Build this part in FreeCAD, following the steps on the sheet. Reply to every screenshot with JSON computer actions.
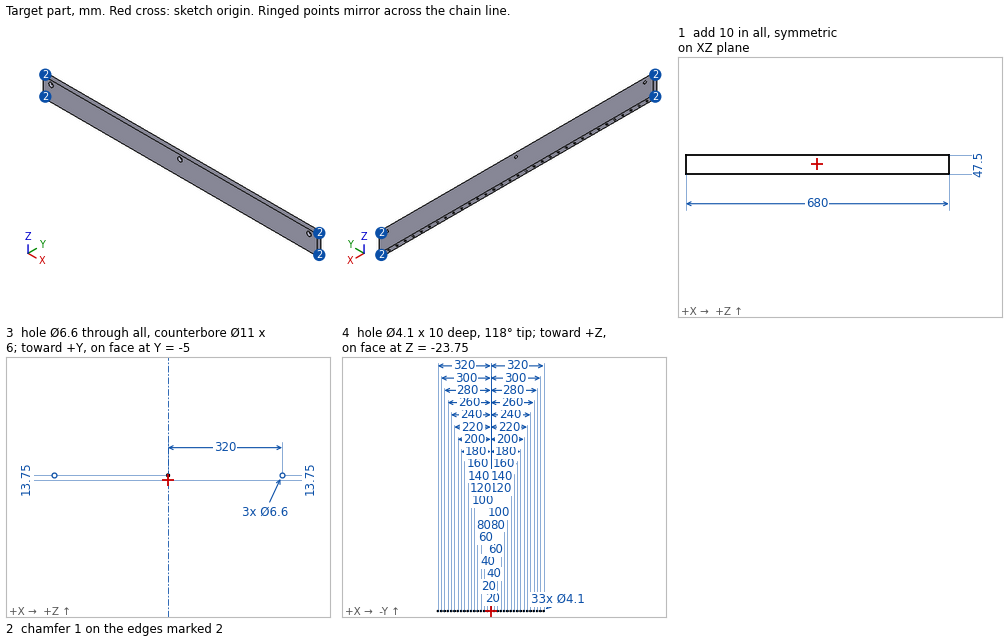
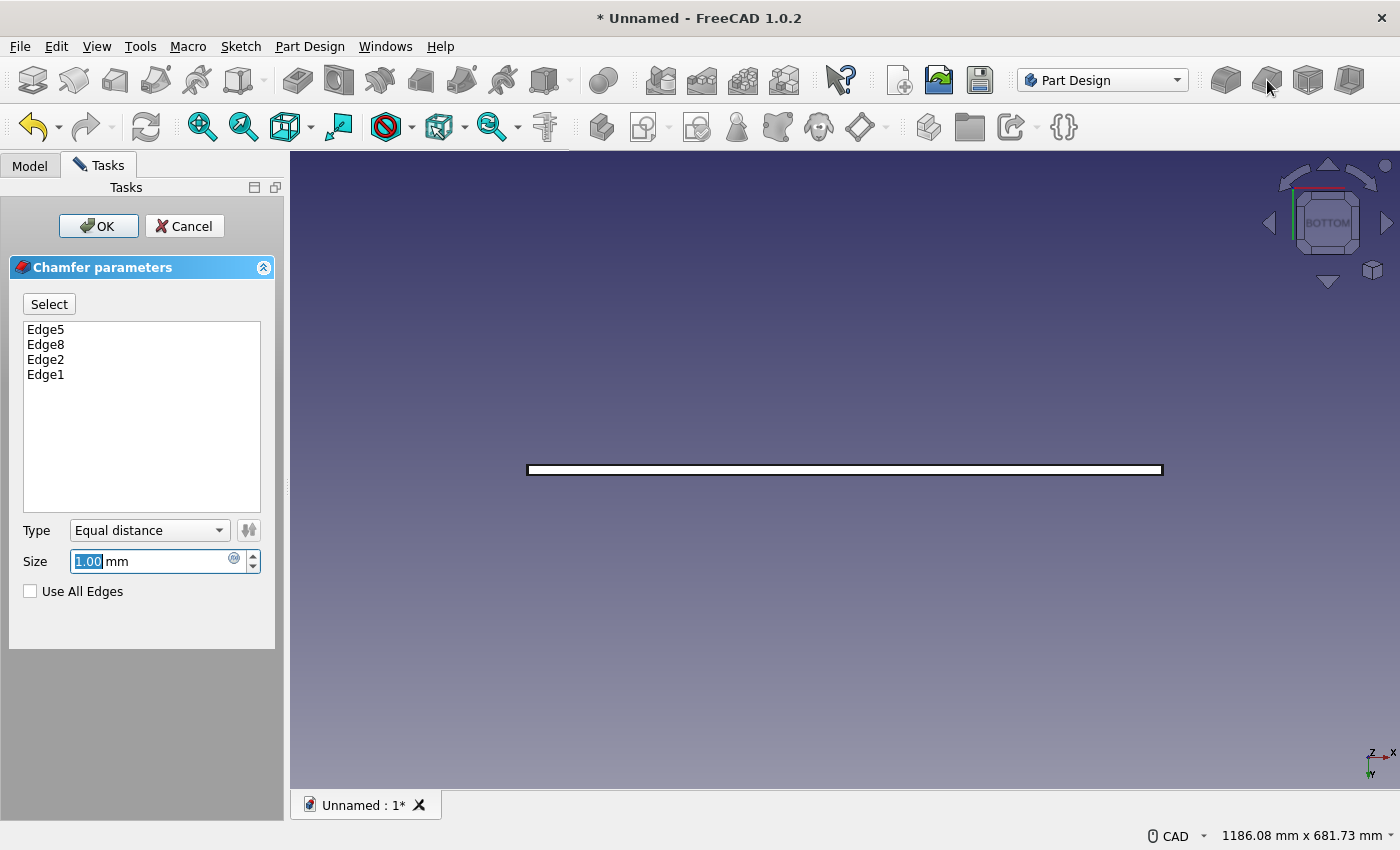
{"action": "type", "text": "1"}
{"action": "key", "text": "Tab"}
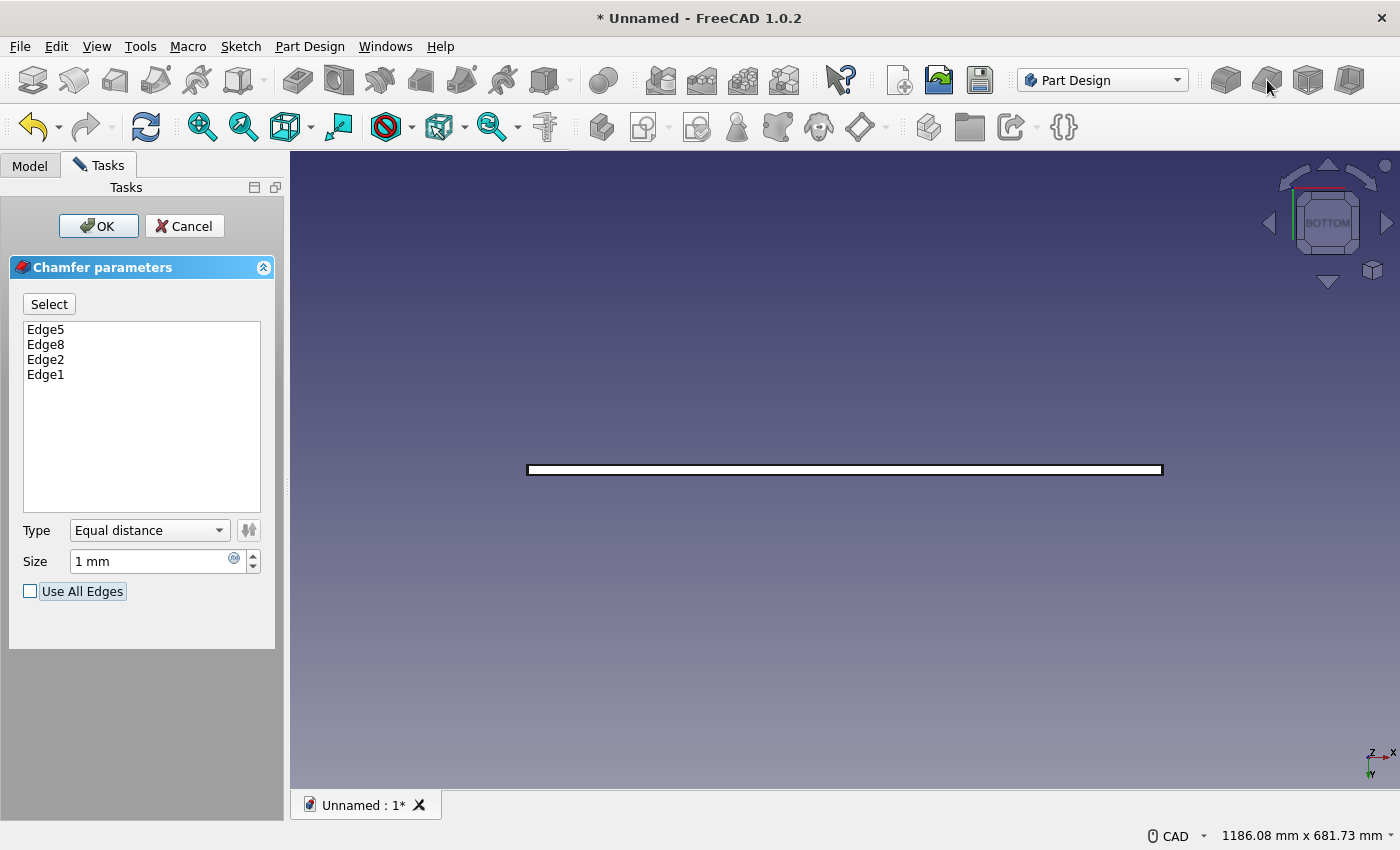
{"action": "left_click", "coordinate": [99, 226]}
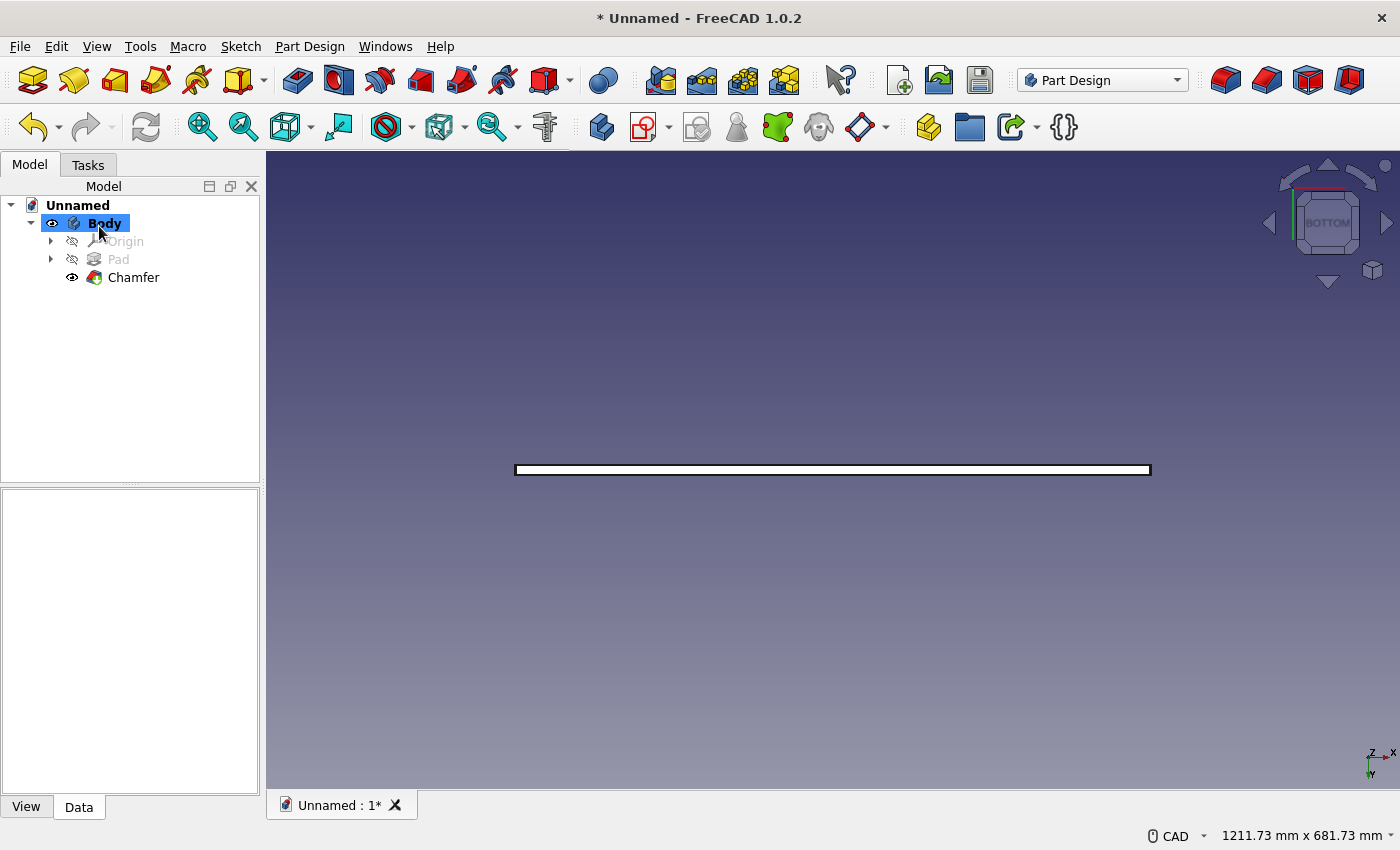
{"action": "key", "text": "0"}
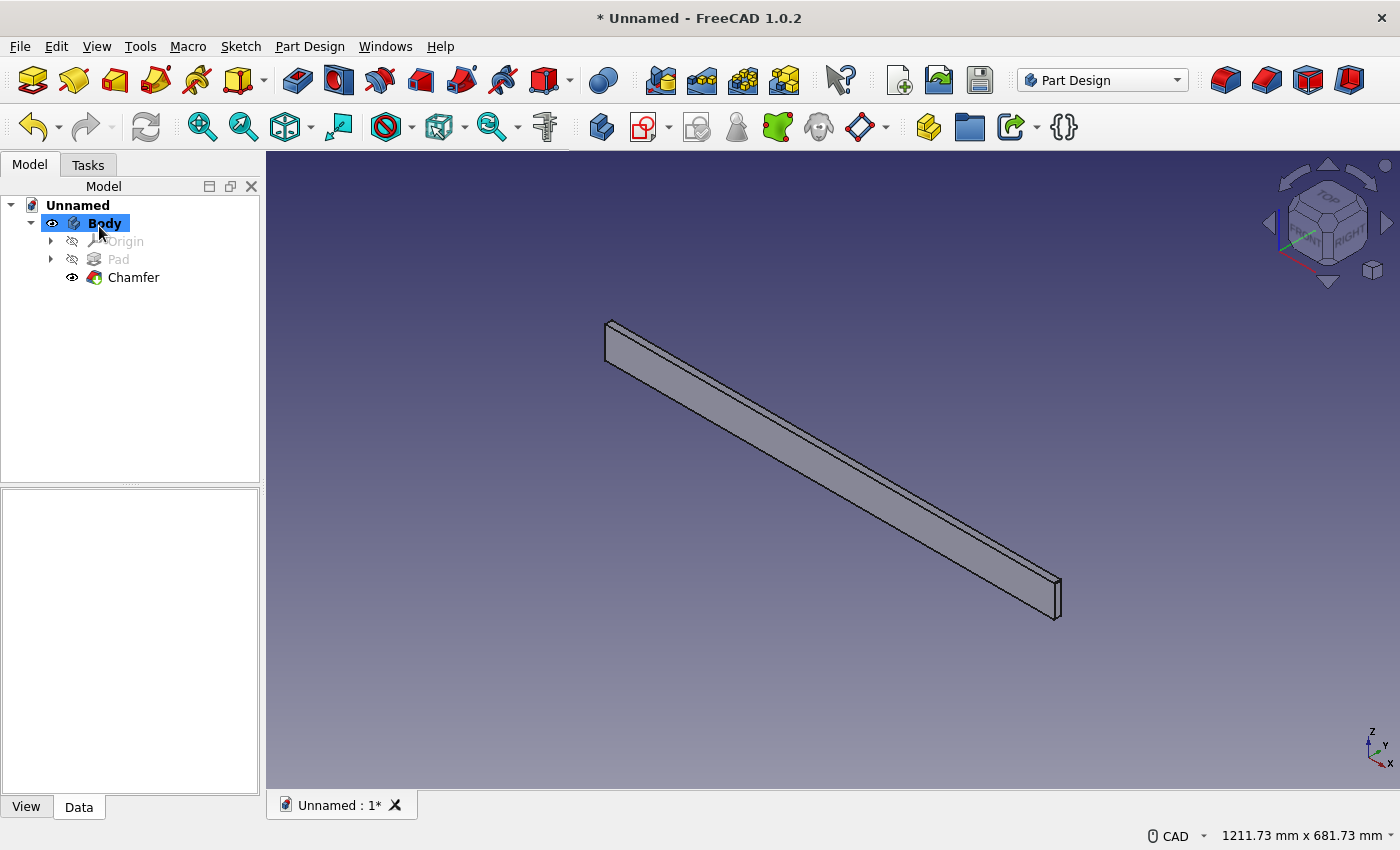
{"action": "left_click", "coordinate": [1023, 582]}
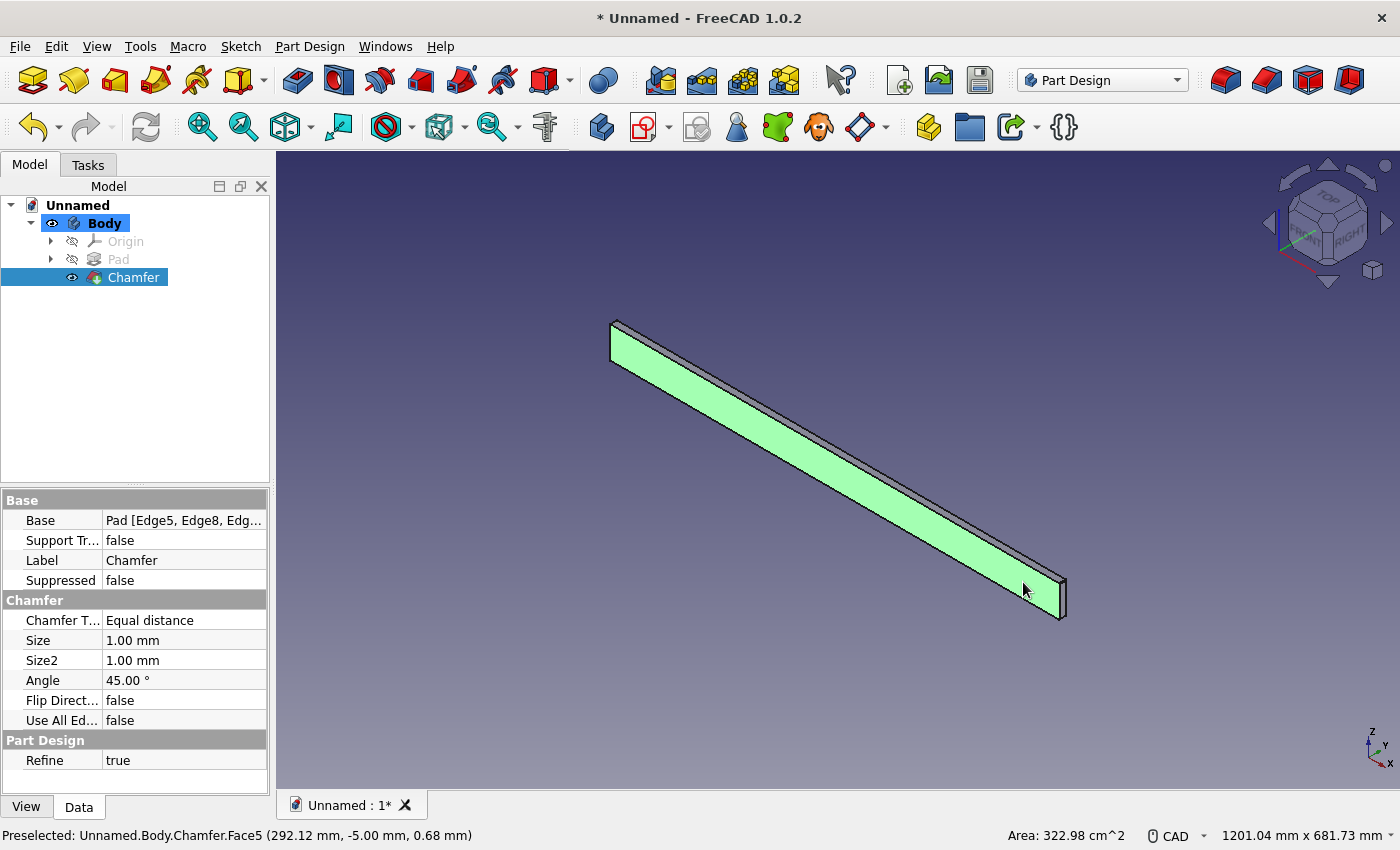
{"action": "left_click", "coordinate": [642, 128]}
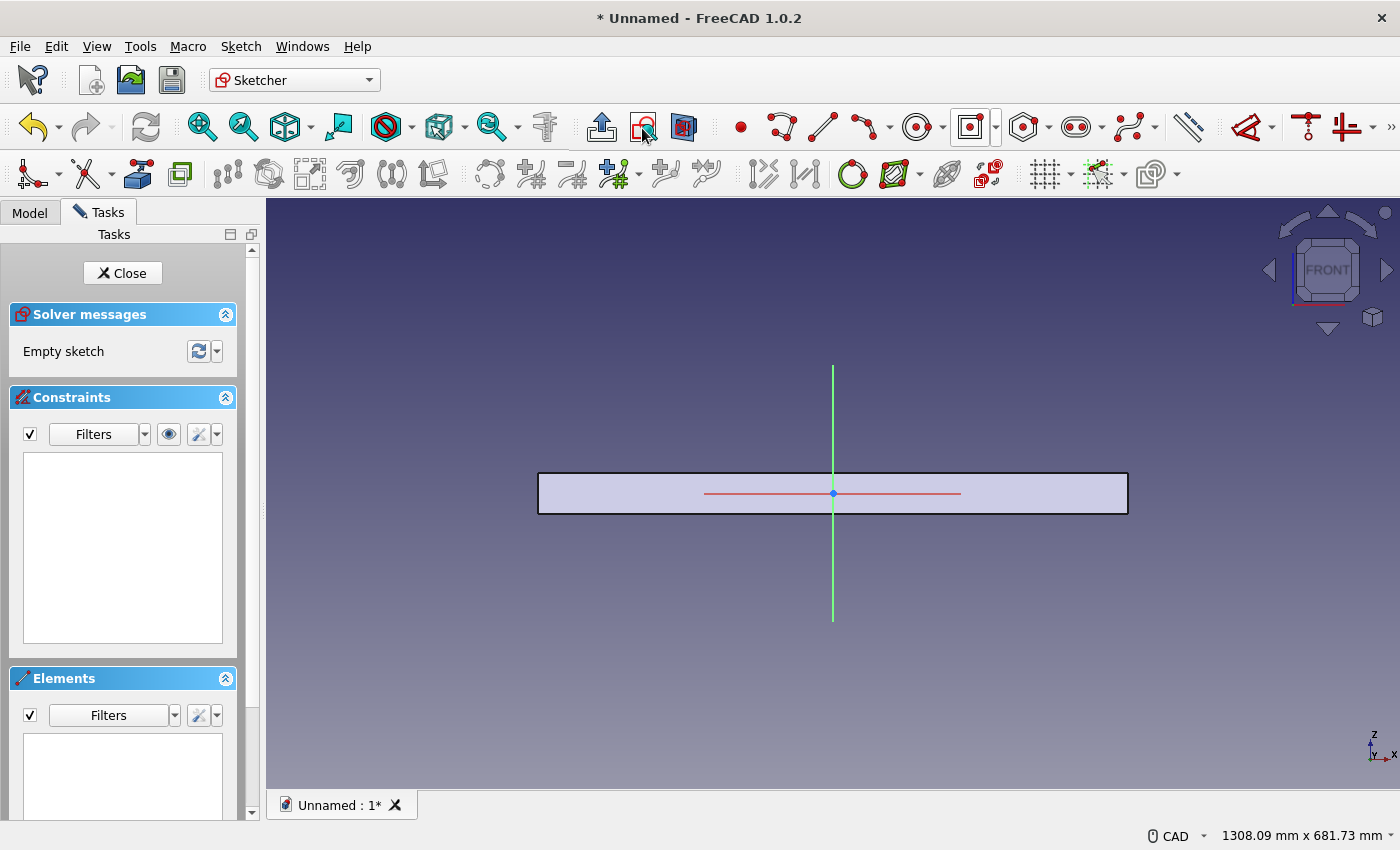
{"action": "left_click", "coordinate": [916, 128]}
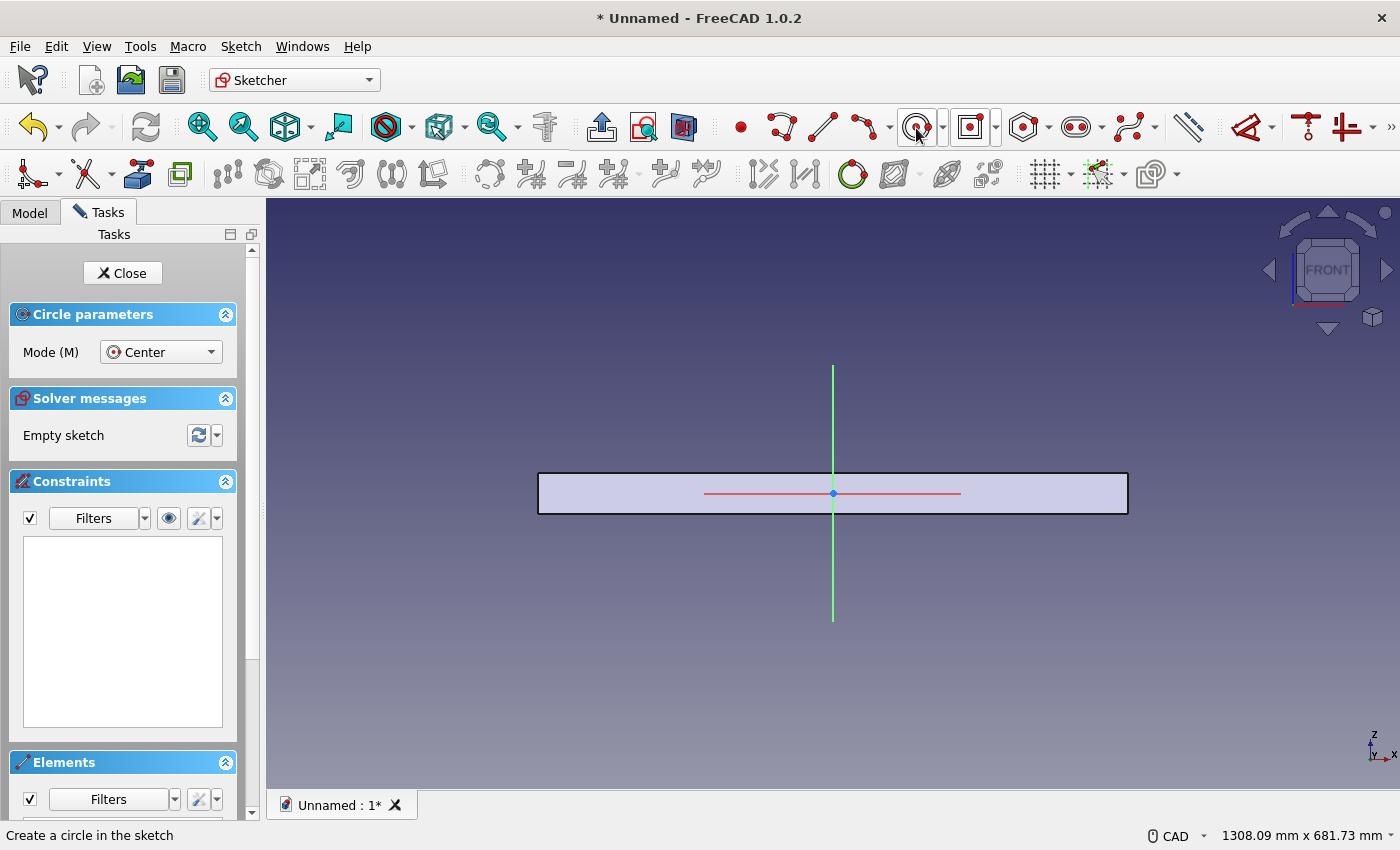
{"action": "scroll", "coordinate": [1110, 482], "scroll_direction": "up", "scroll_amount": 11}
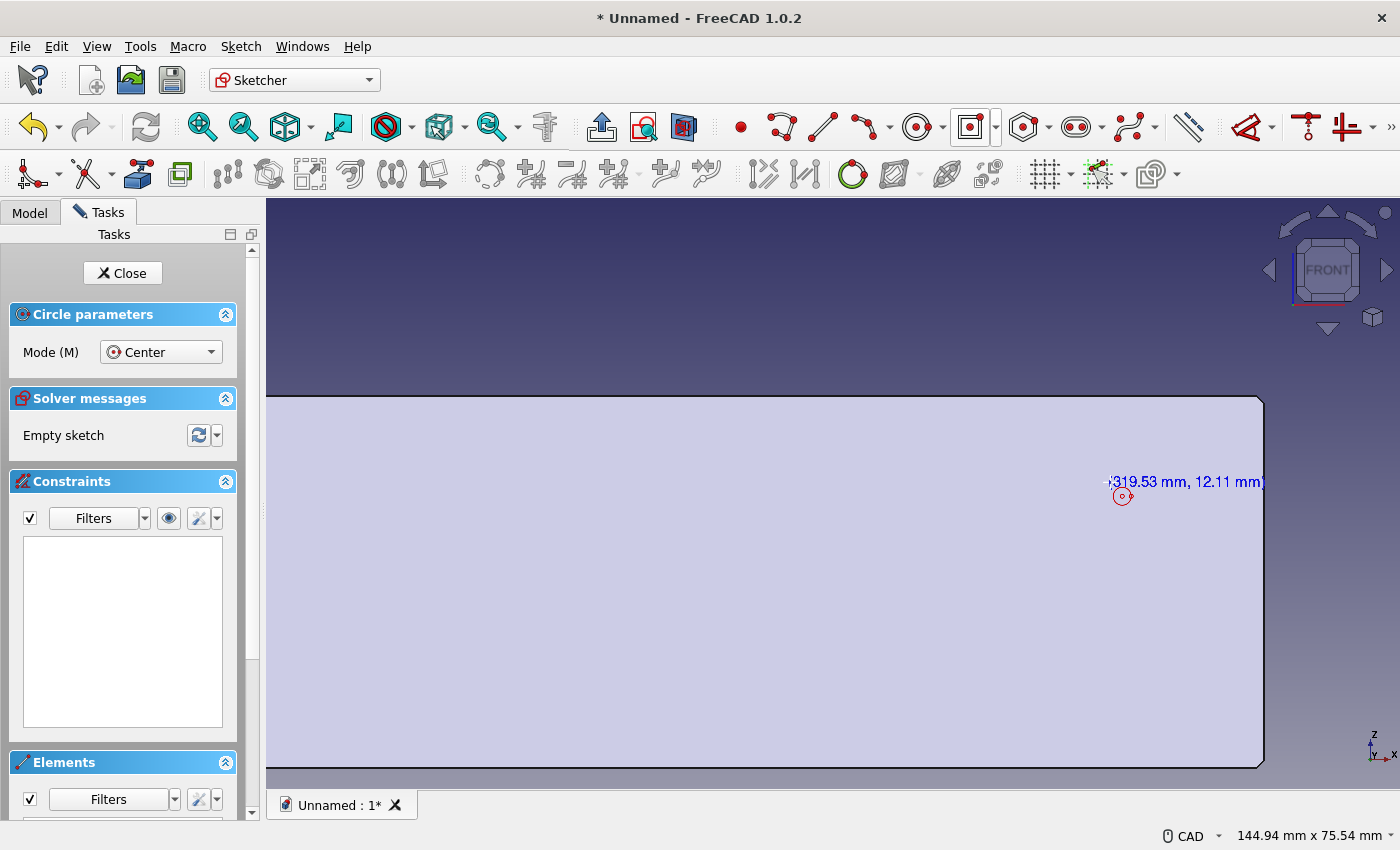
{"action": "scroll", "coordinate": [1103, 490], "scroll_direction": "down", "scroll_amount": 10}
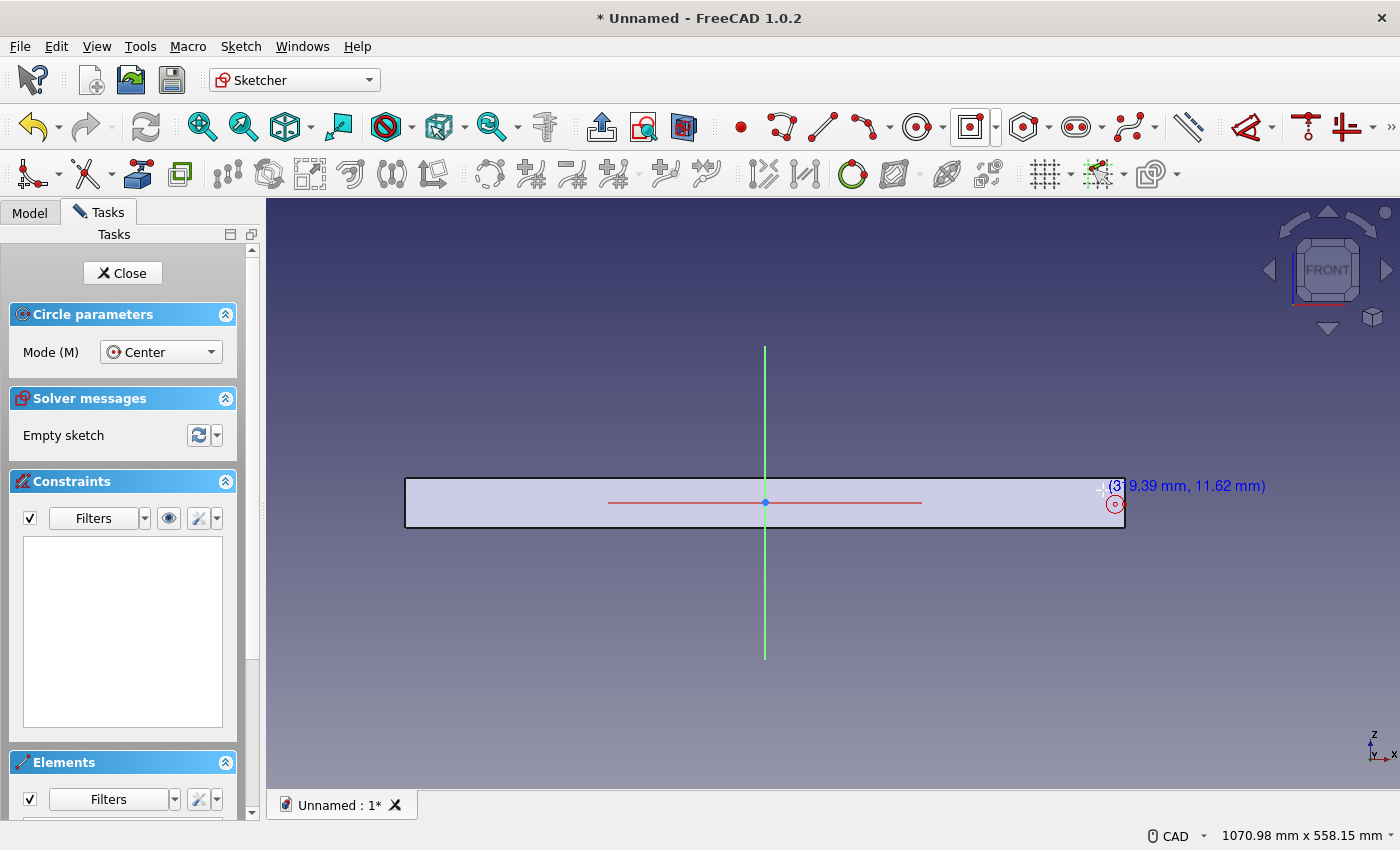
{"action": "left_click", "coordinate": [1104, 488]}
{"action": "mouse_move", "coordinate": [1107, 486]}